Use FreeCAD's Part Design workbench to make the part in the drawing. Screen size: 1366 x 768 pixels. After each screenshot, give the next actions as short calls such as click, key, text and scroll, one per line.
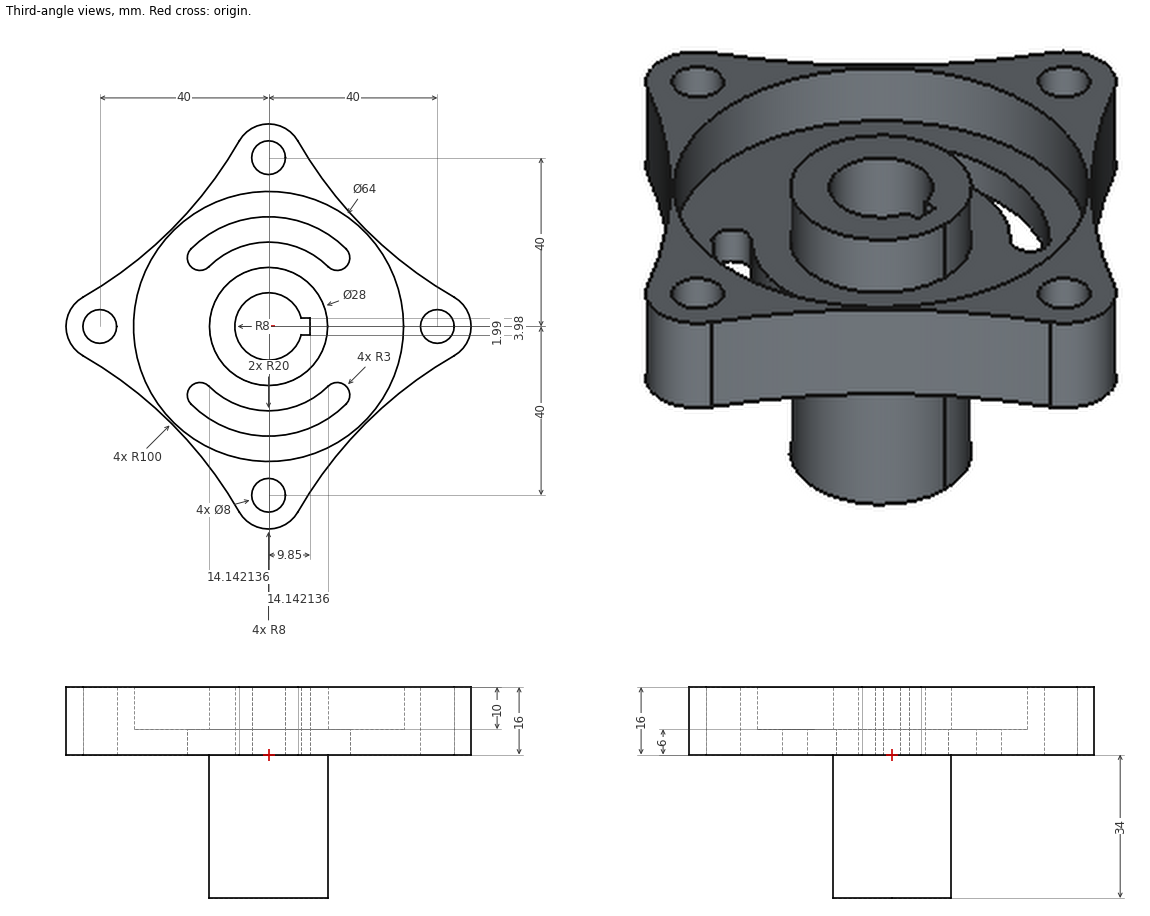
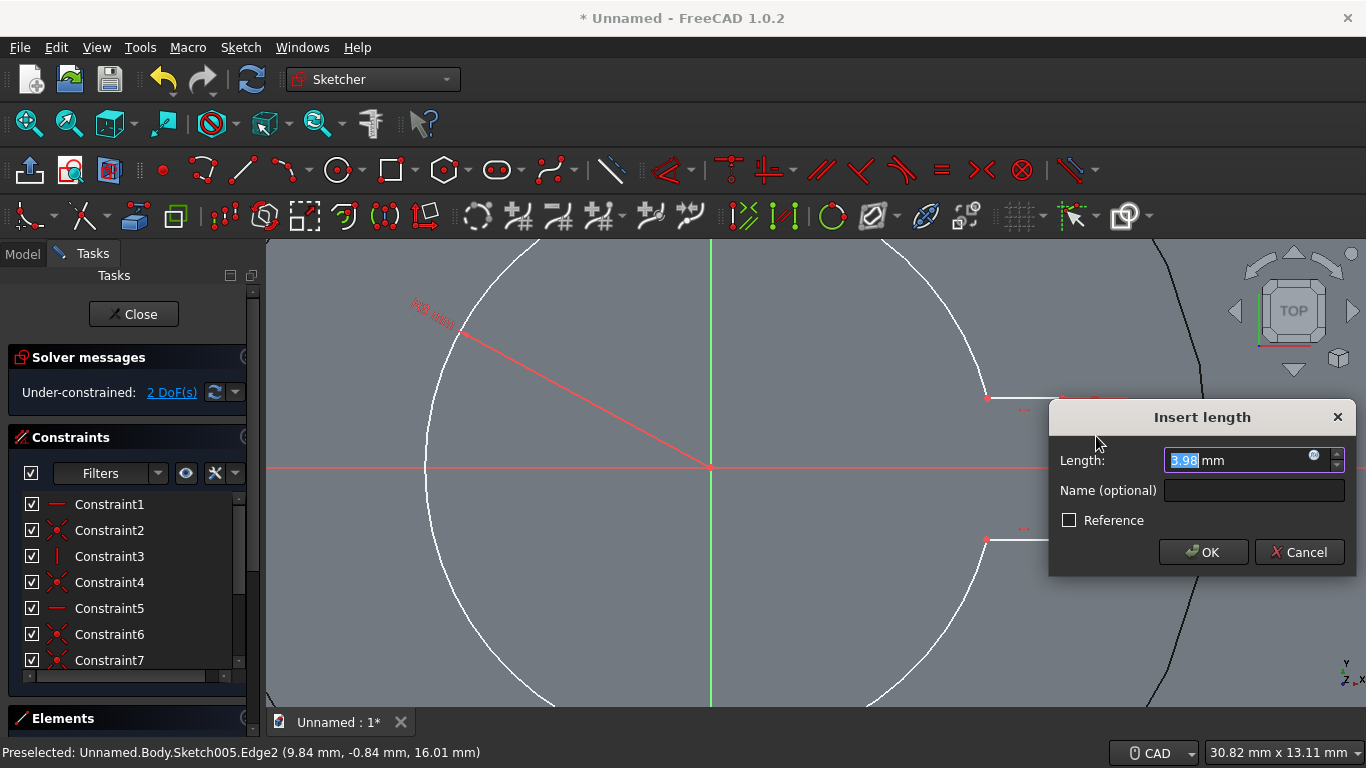
text(3.98)
key(Return)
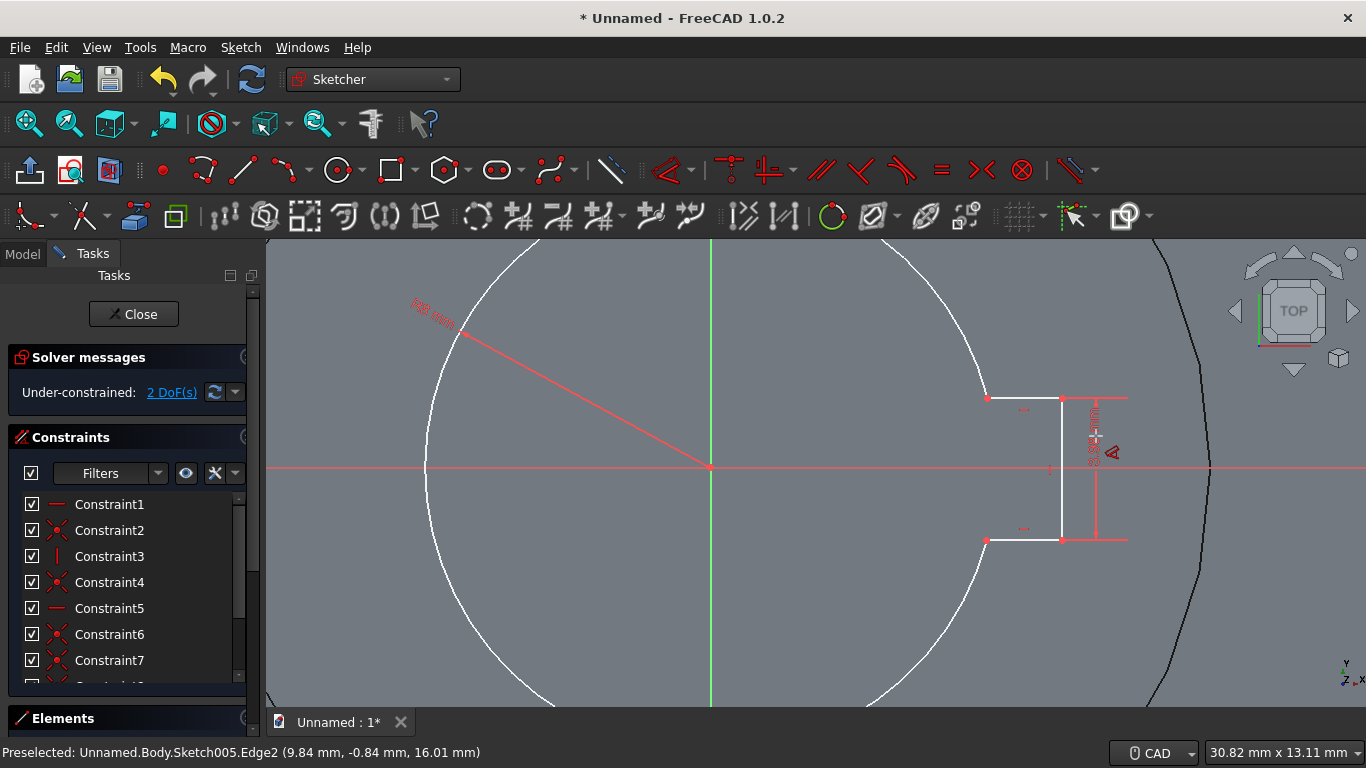
click(987, 540)
click(1021, 504)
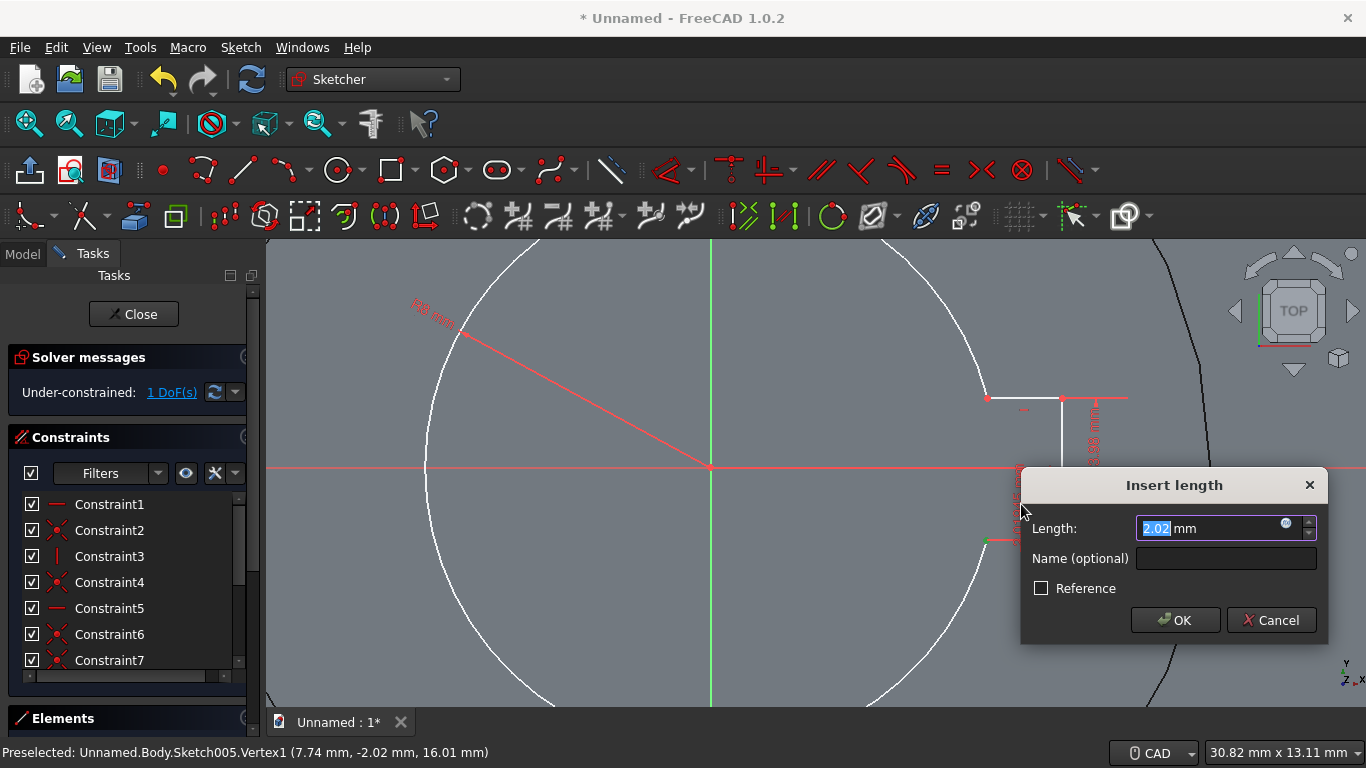
text(1.99)
key(Return)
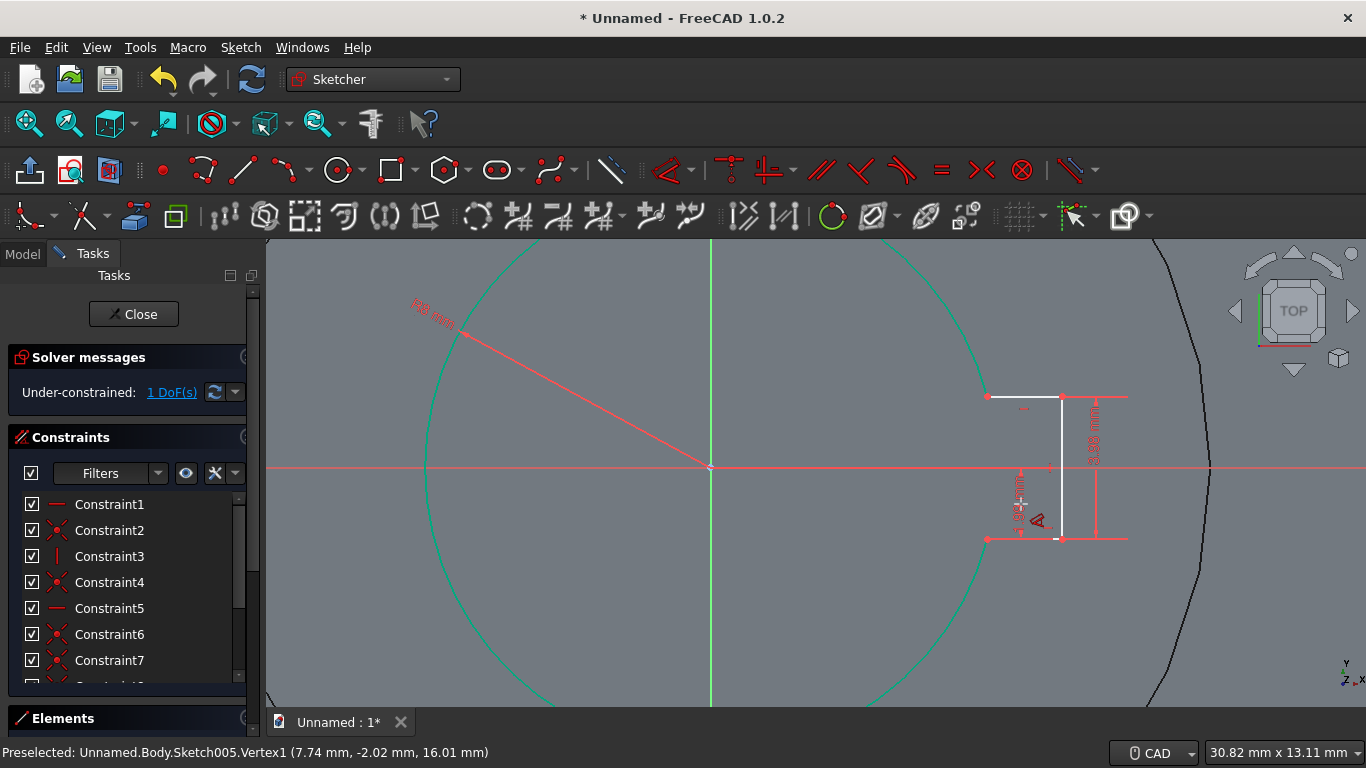
click(1062, 539)
click(886, 573)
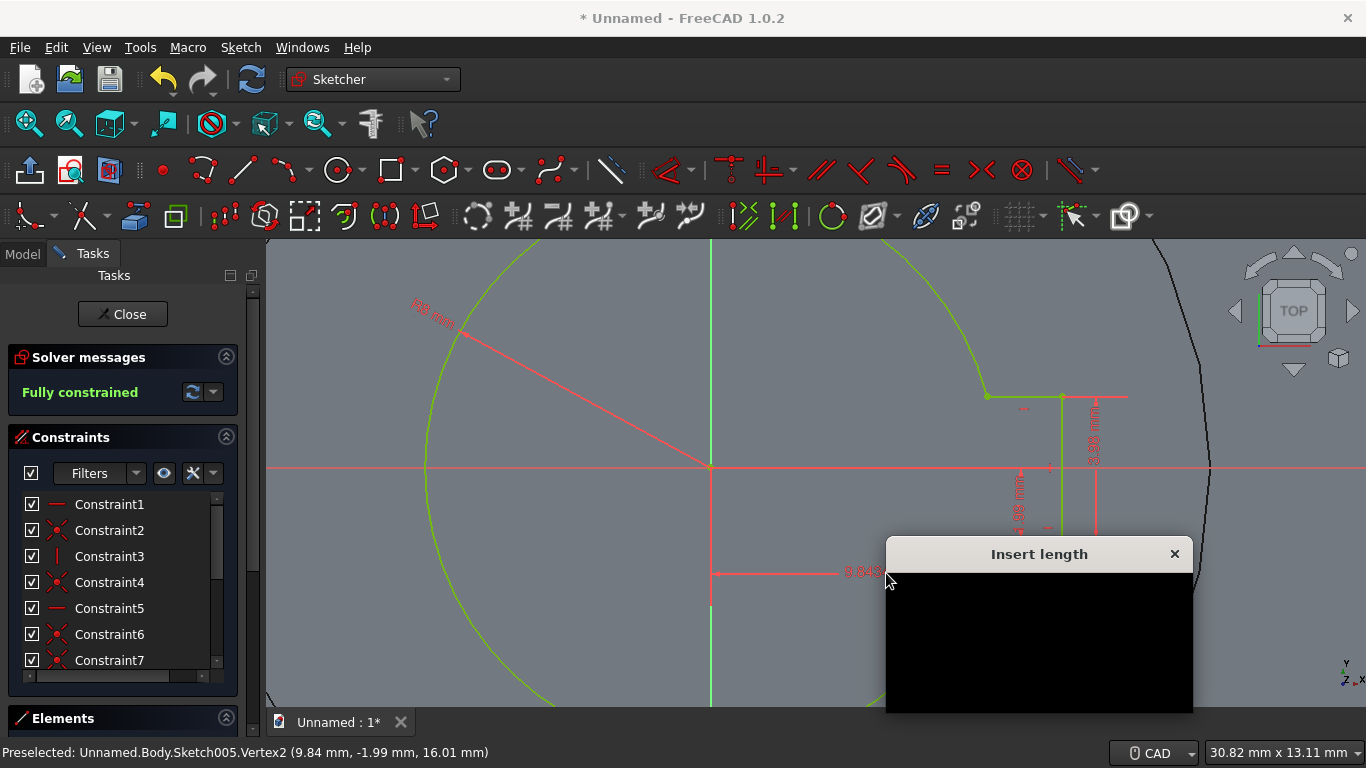
text(9.85)
key(Return)
key(Escape)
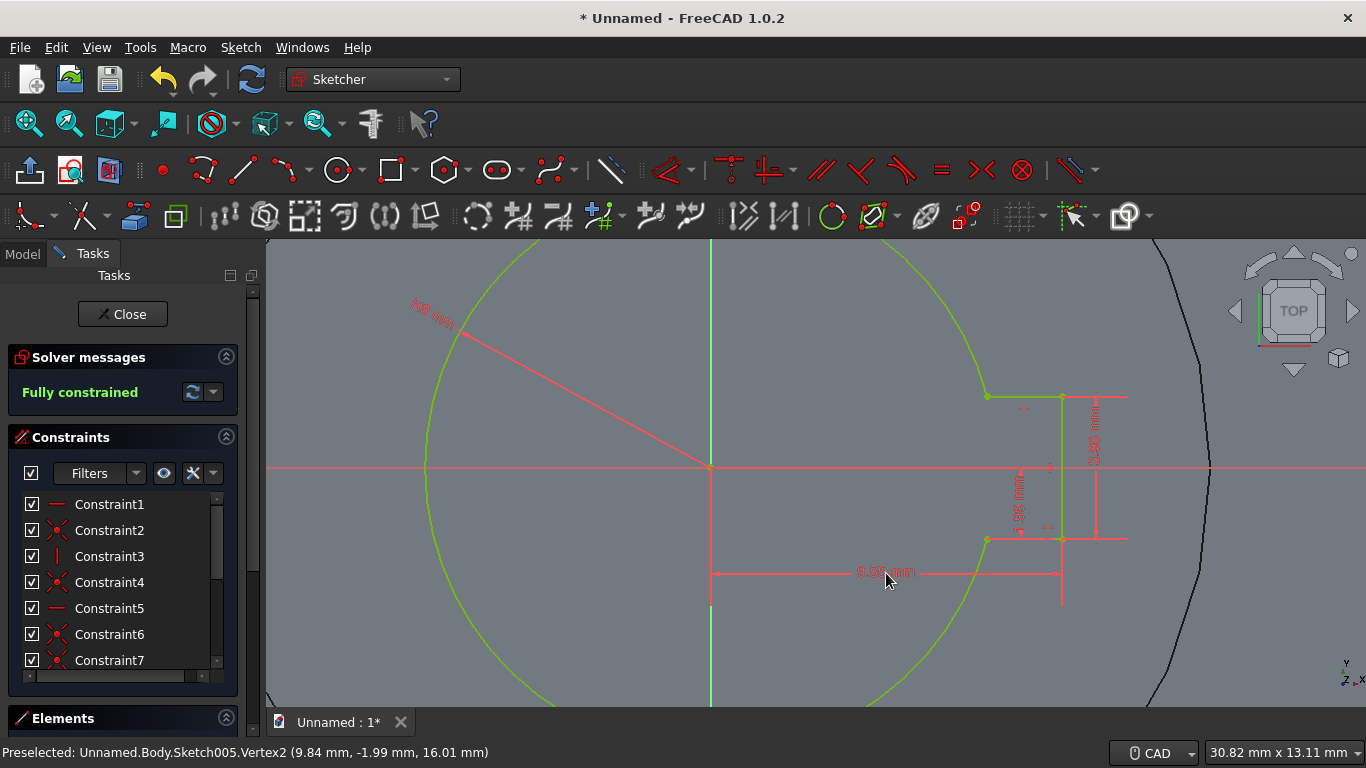
click(123, 314)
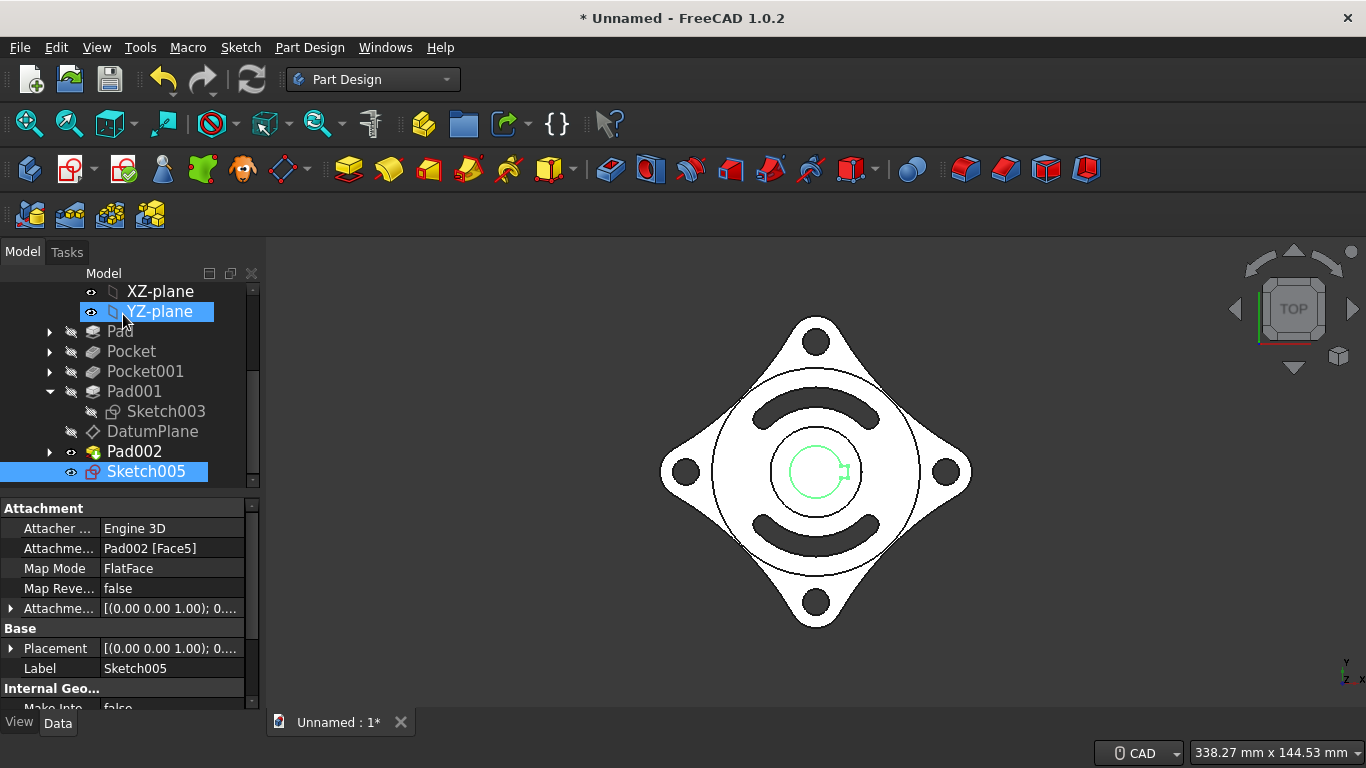
click(612, 170)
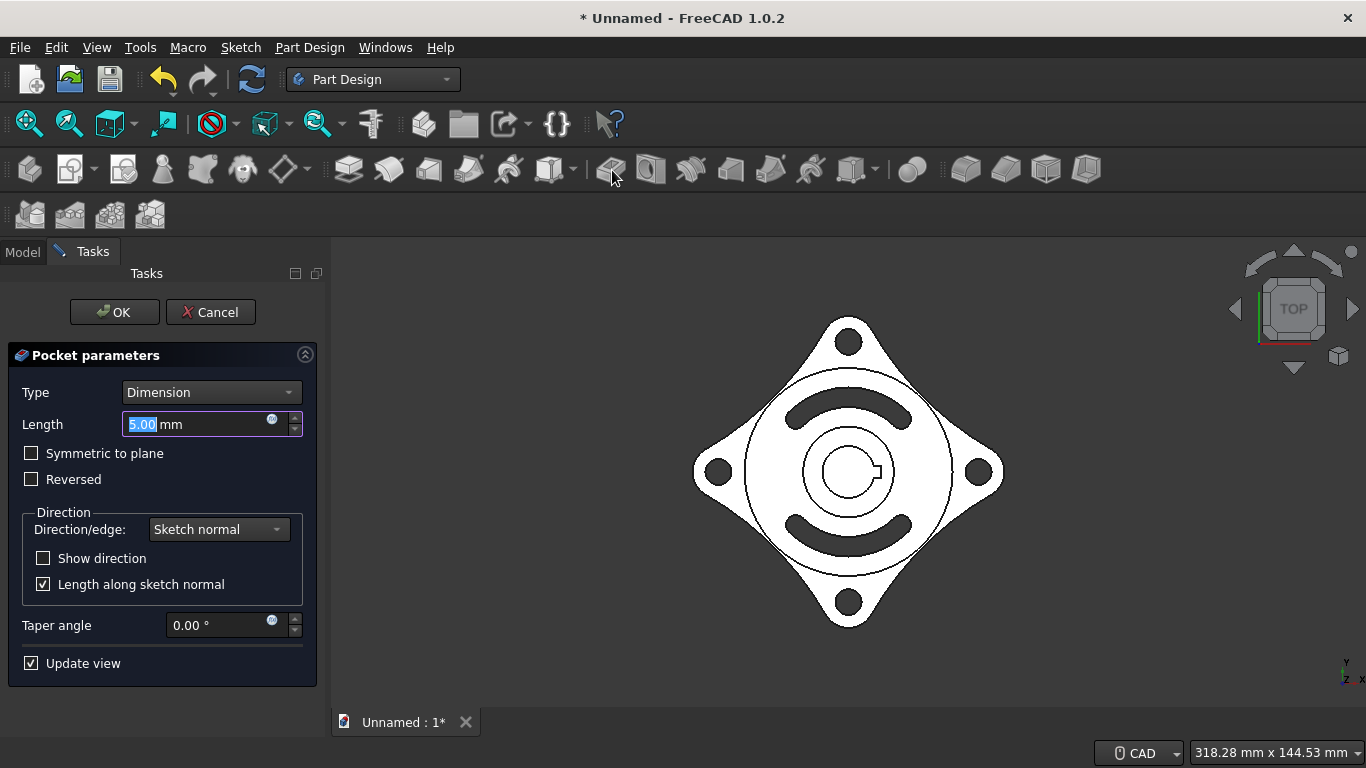
text(16)
key(Tab)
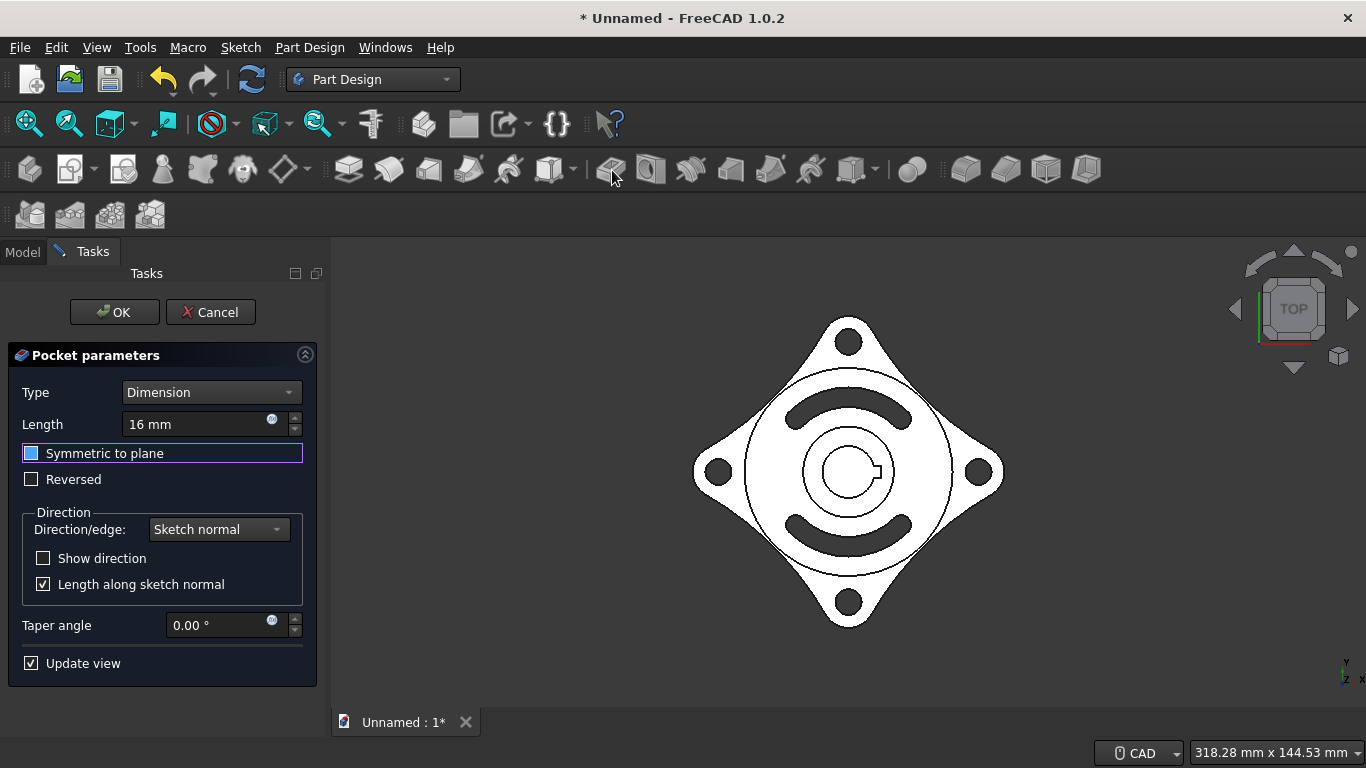
click(115, 312)